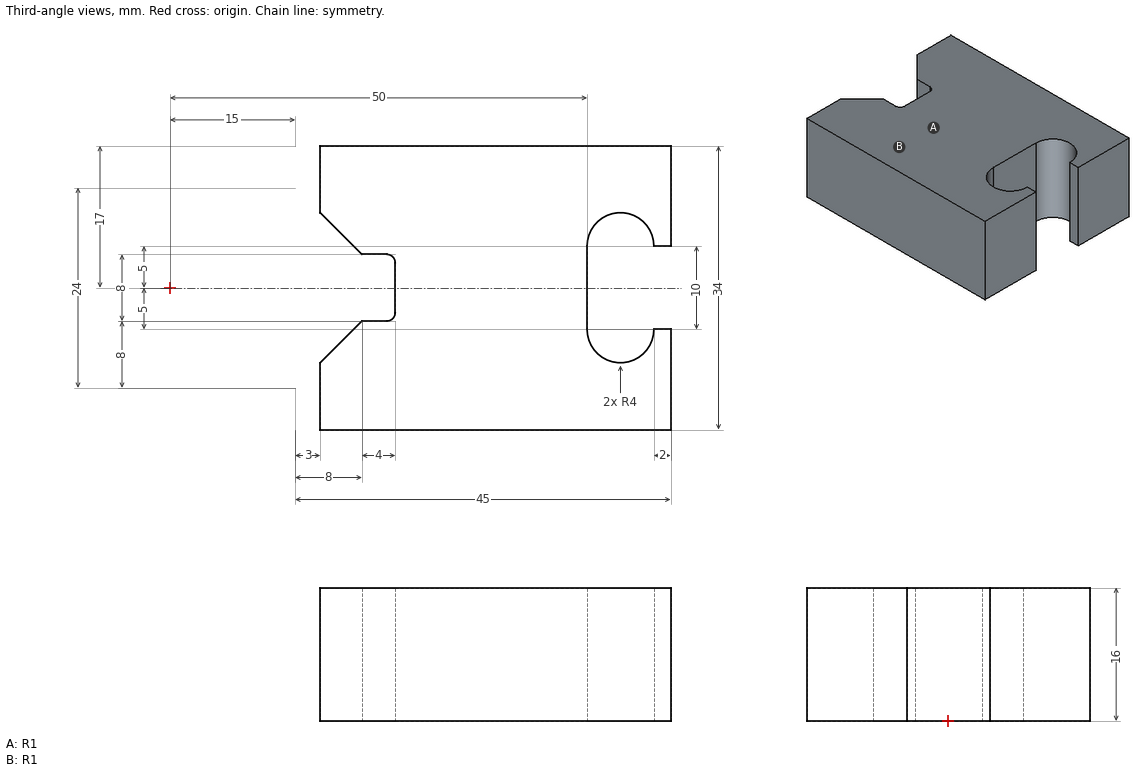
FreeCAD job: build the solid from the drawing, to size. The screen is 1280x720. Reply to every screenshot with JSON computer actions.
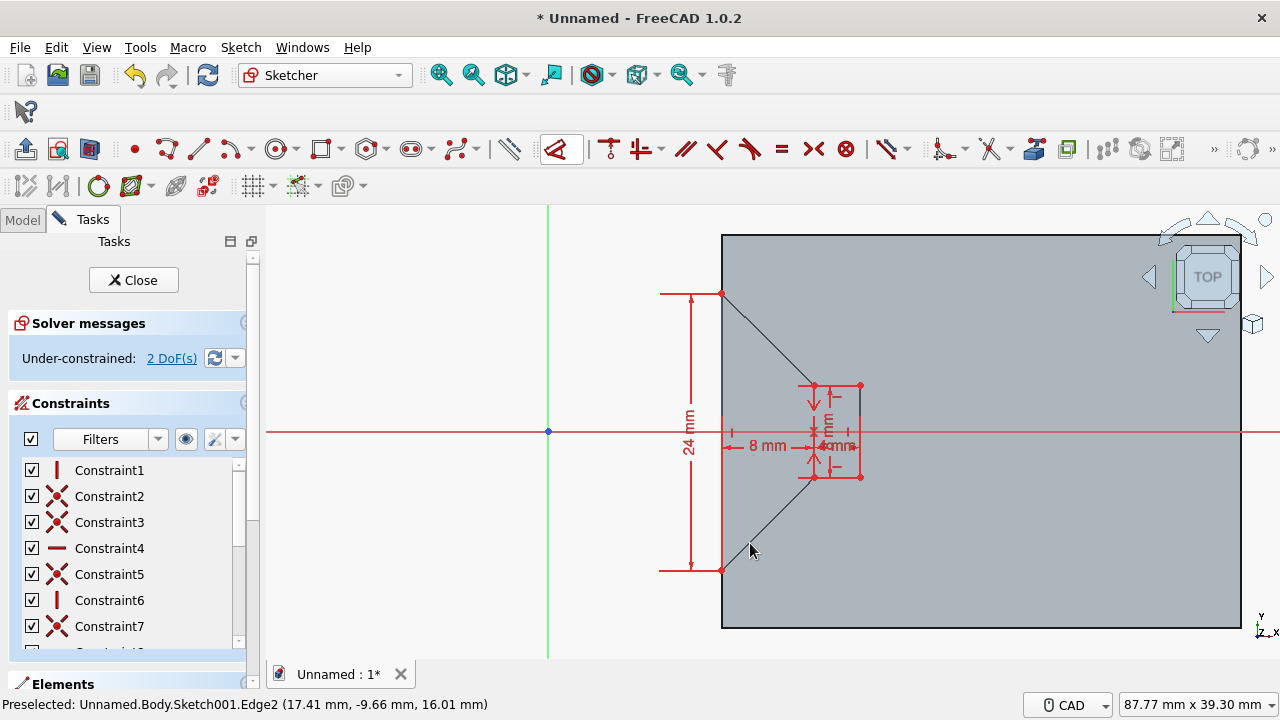
{"action": "left_click", "coordinate": [749, 543]}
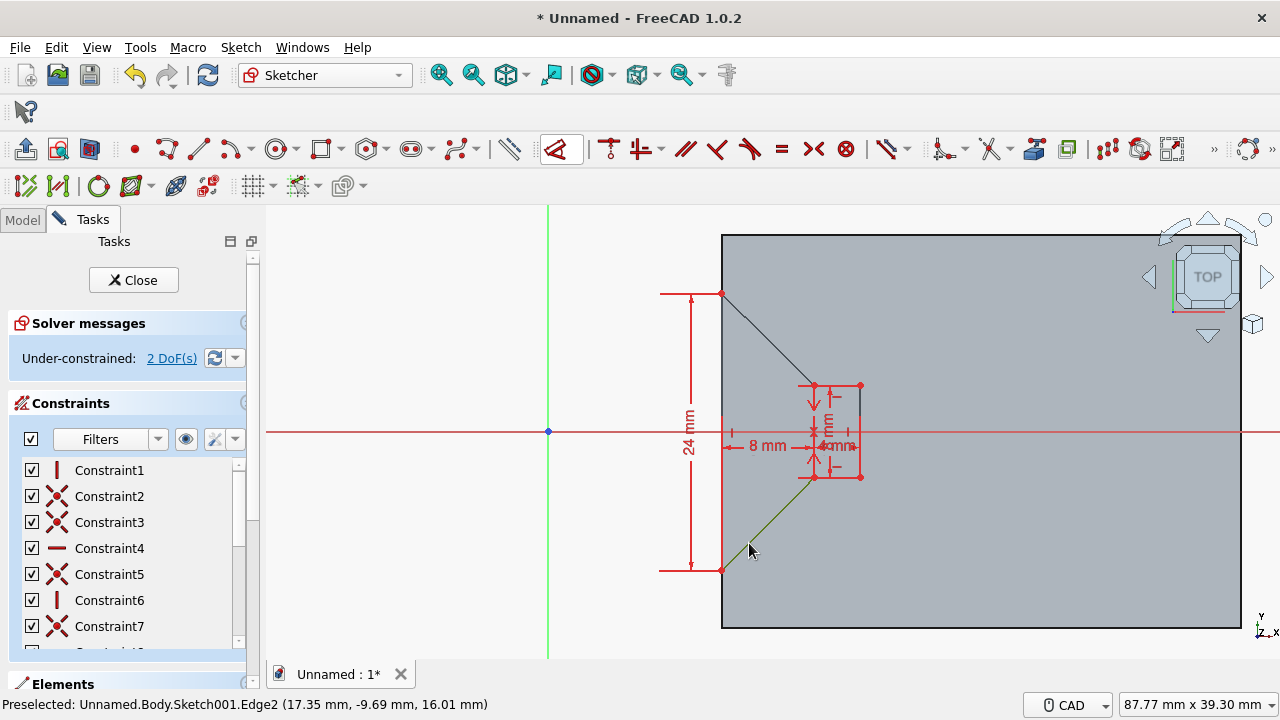
{"action": "key", "text": "i"}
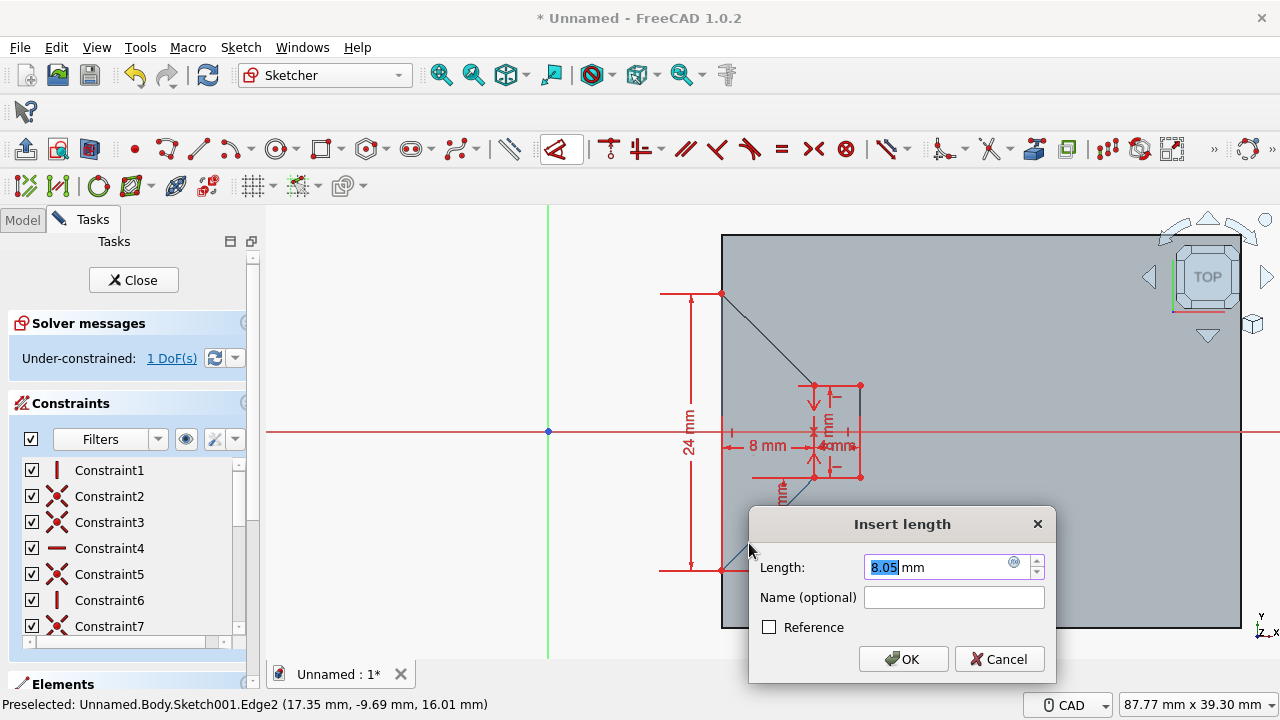
{"action": "type", "text": "8"}
{"action": "key", "text": "Return"}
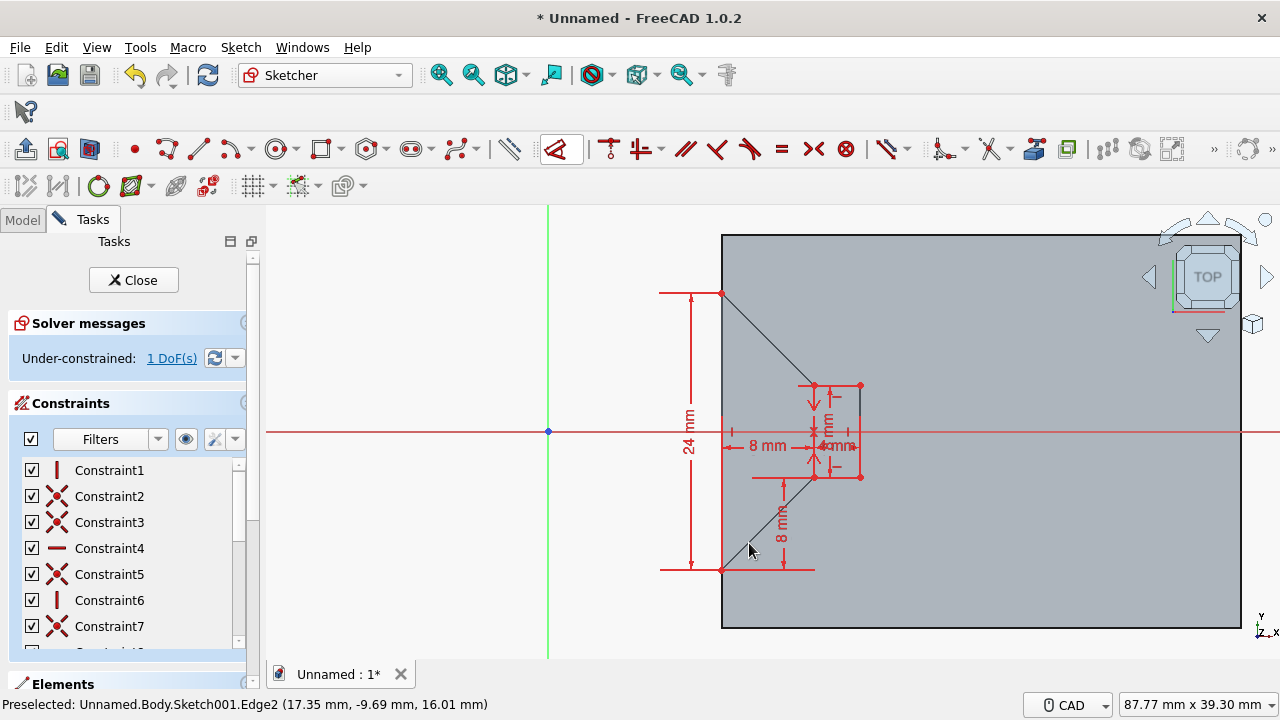
{"action": "left_click", "coordinate": [722, 293]}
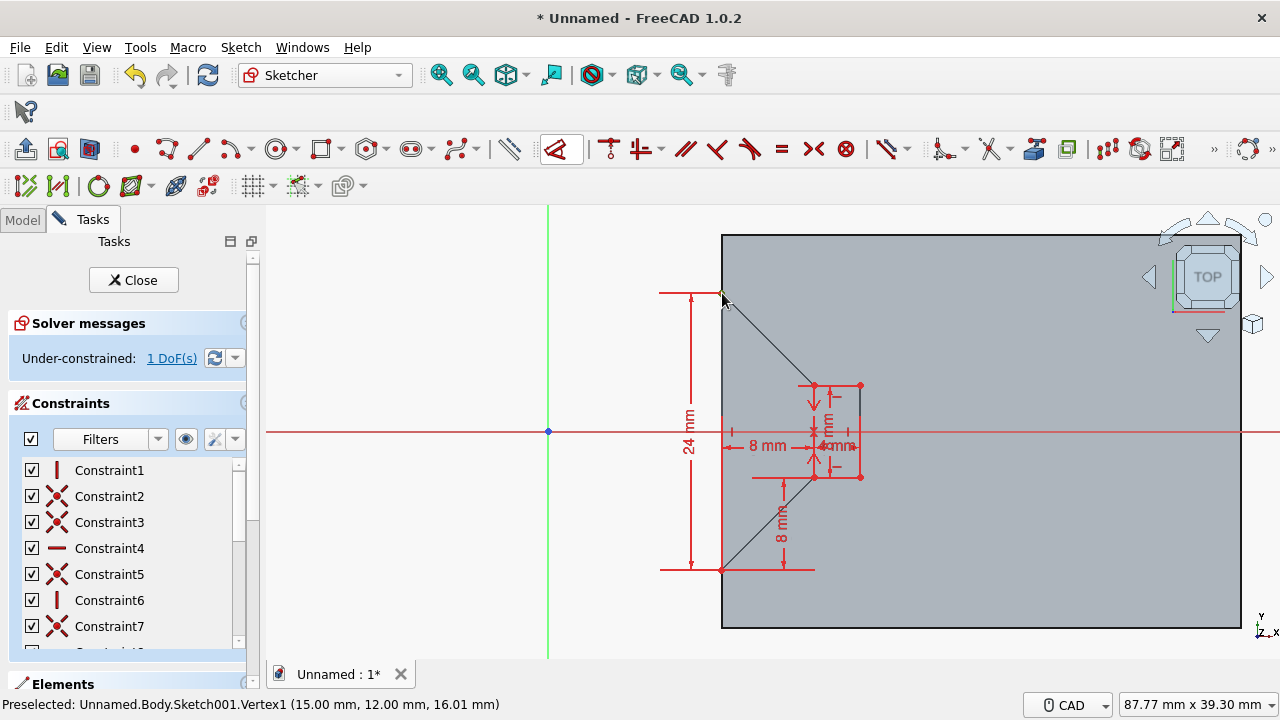
{"action": "key", "text": "l"}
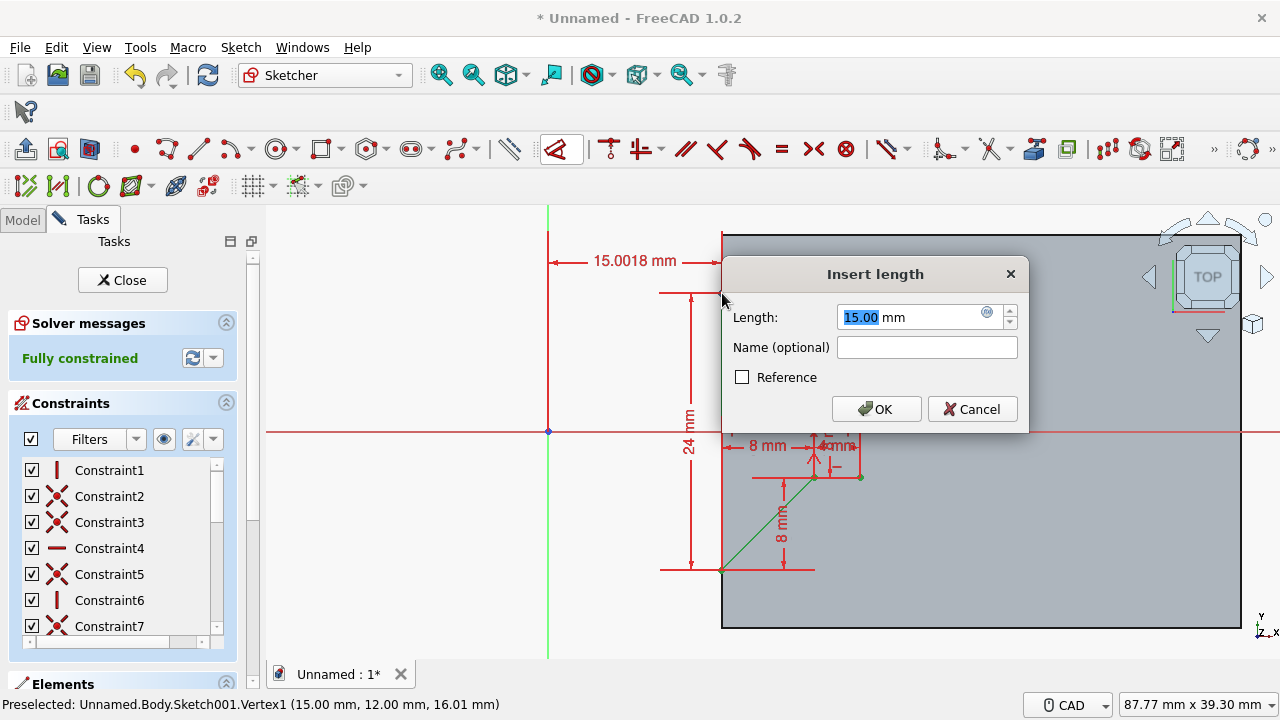
{"action": "type", "text": "15"}
{"action": "key", "text": "Return"}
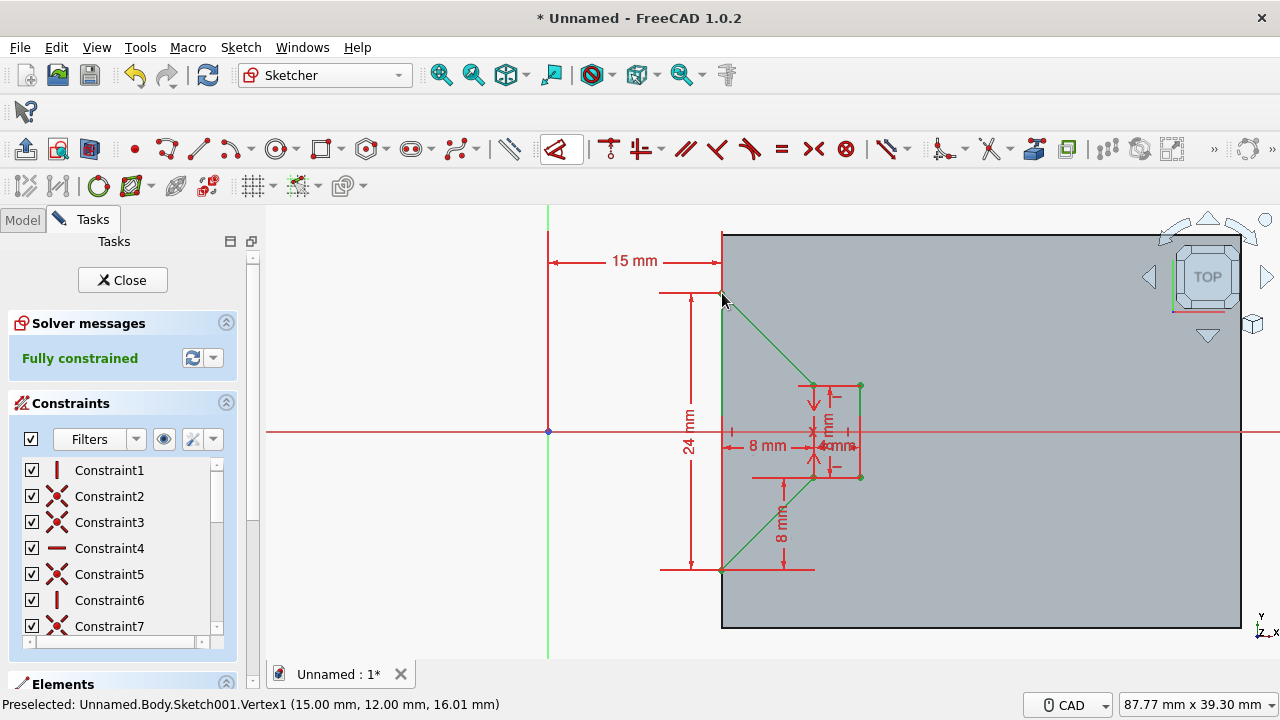
{"action": "left_click", "coordinate": [123, 280]}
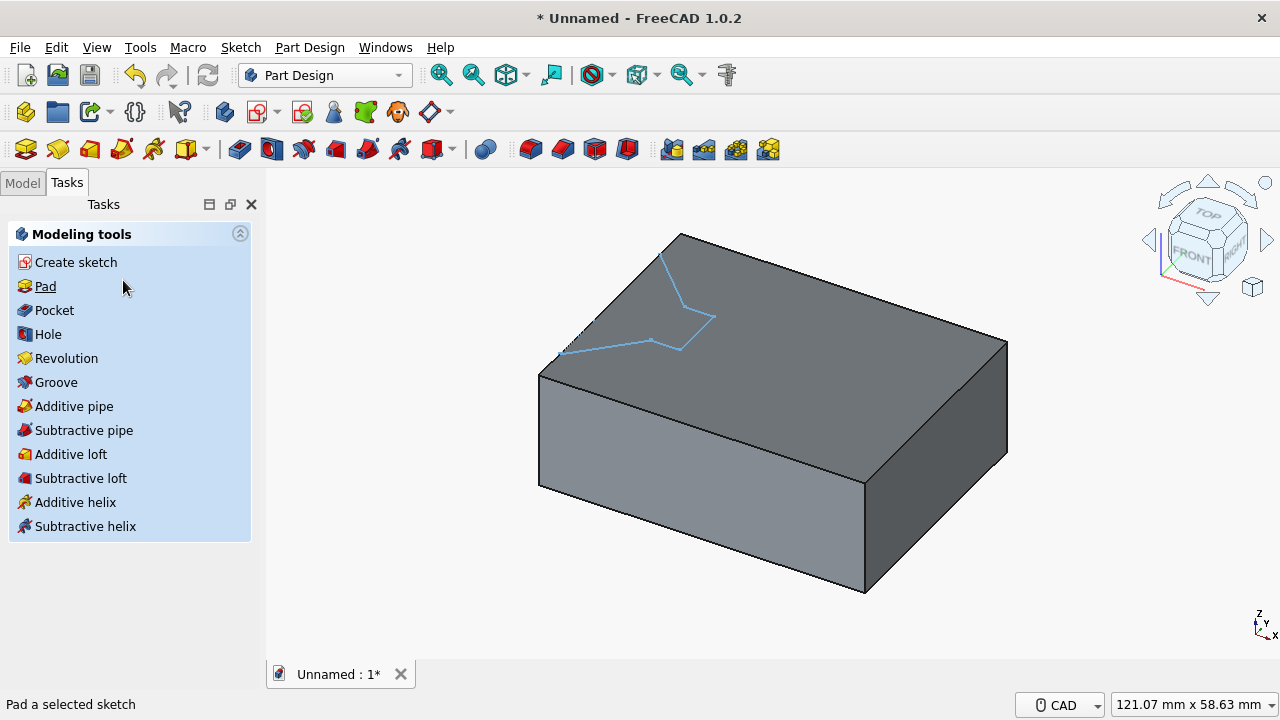
{"action": "left_click", "coordinate": [240, 150]}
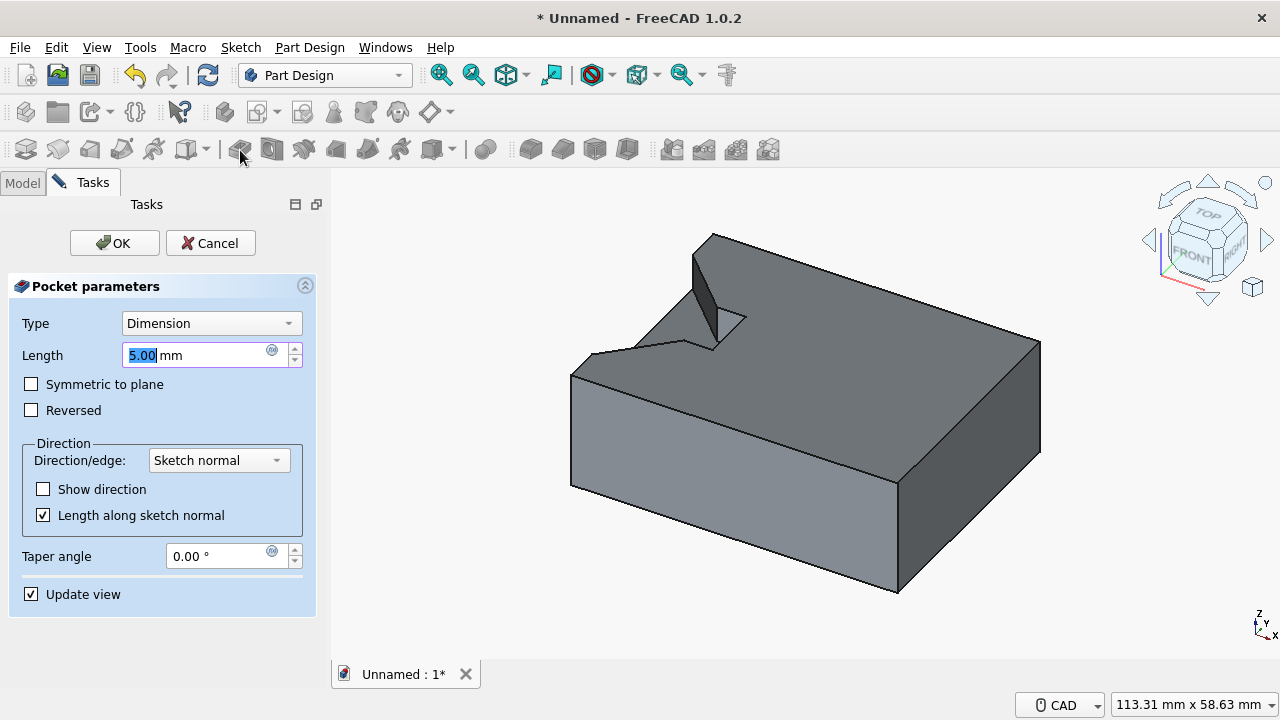
{"action": "left_click", "coordinate": [212, 324]}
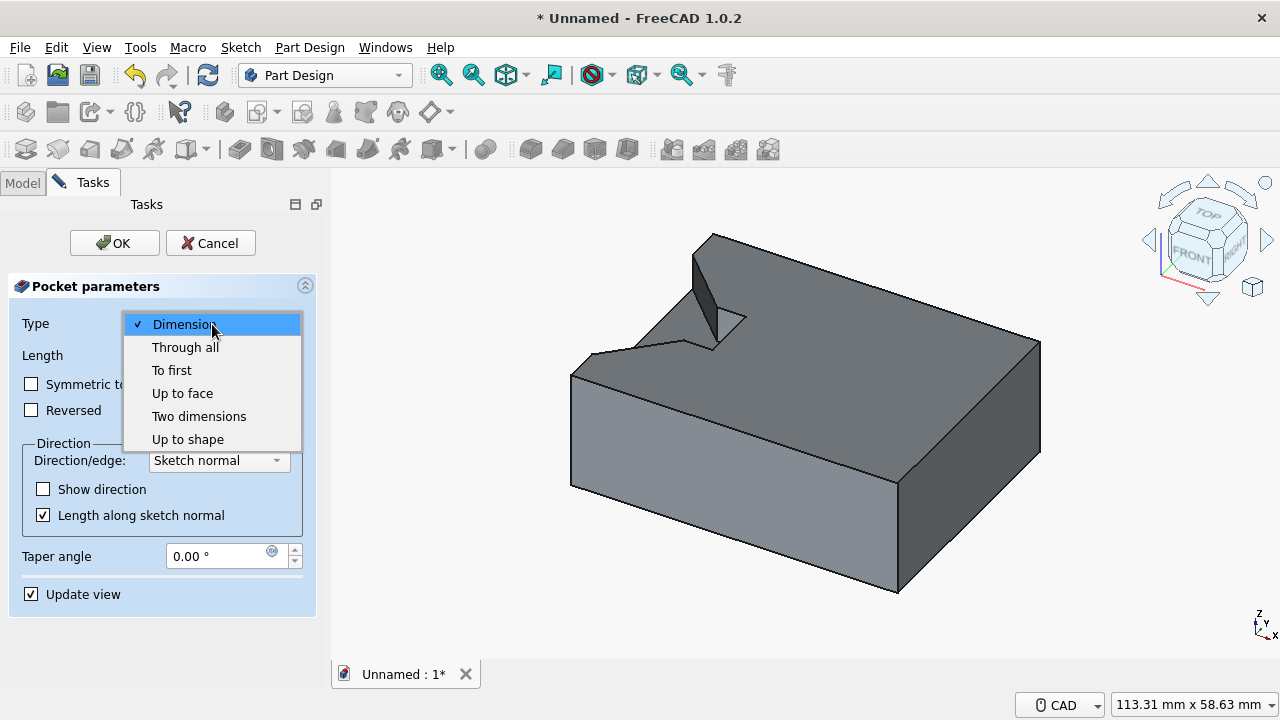
{"action": "left_click", "coordinate": [212, 348]}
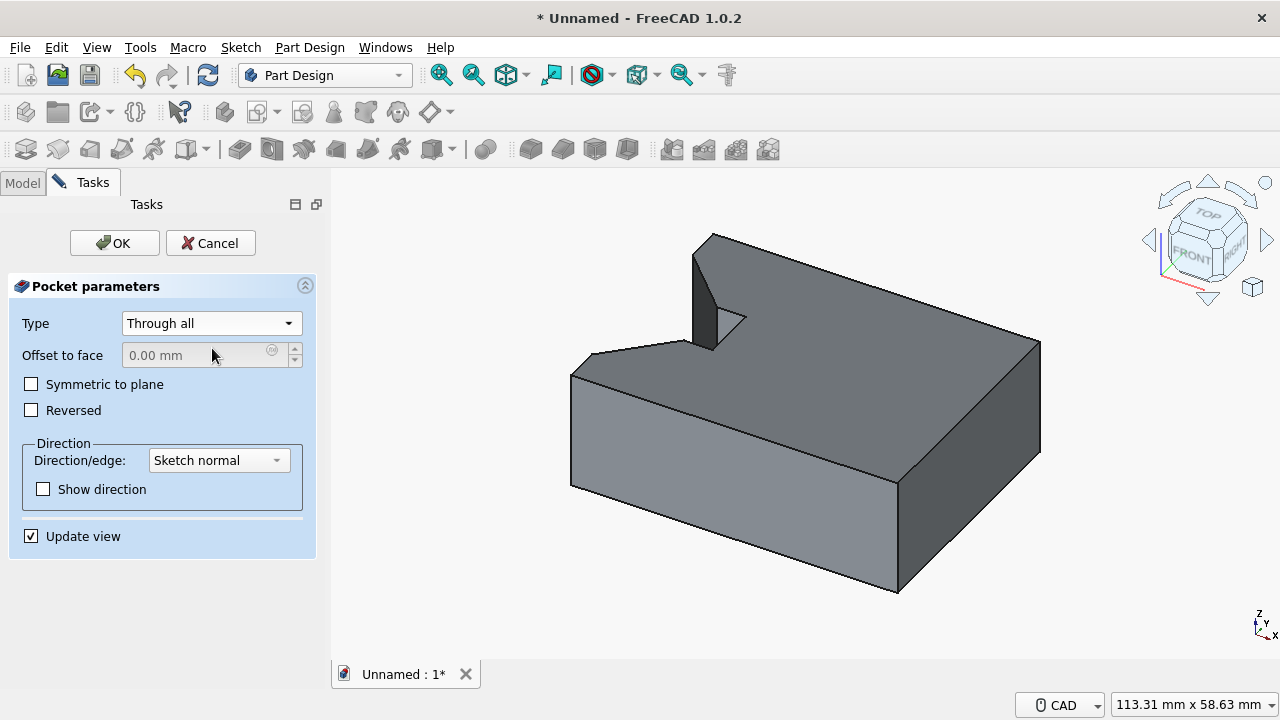
{"action": "left_click", "coordinate": [115, 243]}